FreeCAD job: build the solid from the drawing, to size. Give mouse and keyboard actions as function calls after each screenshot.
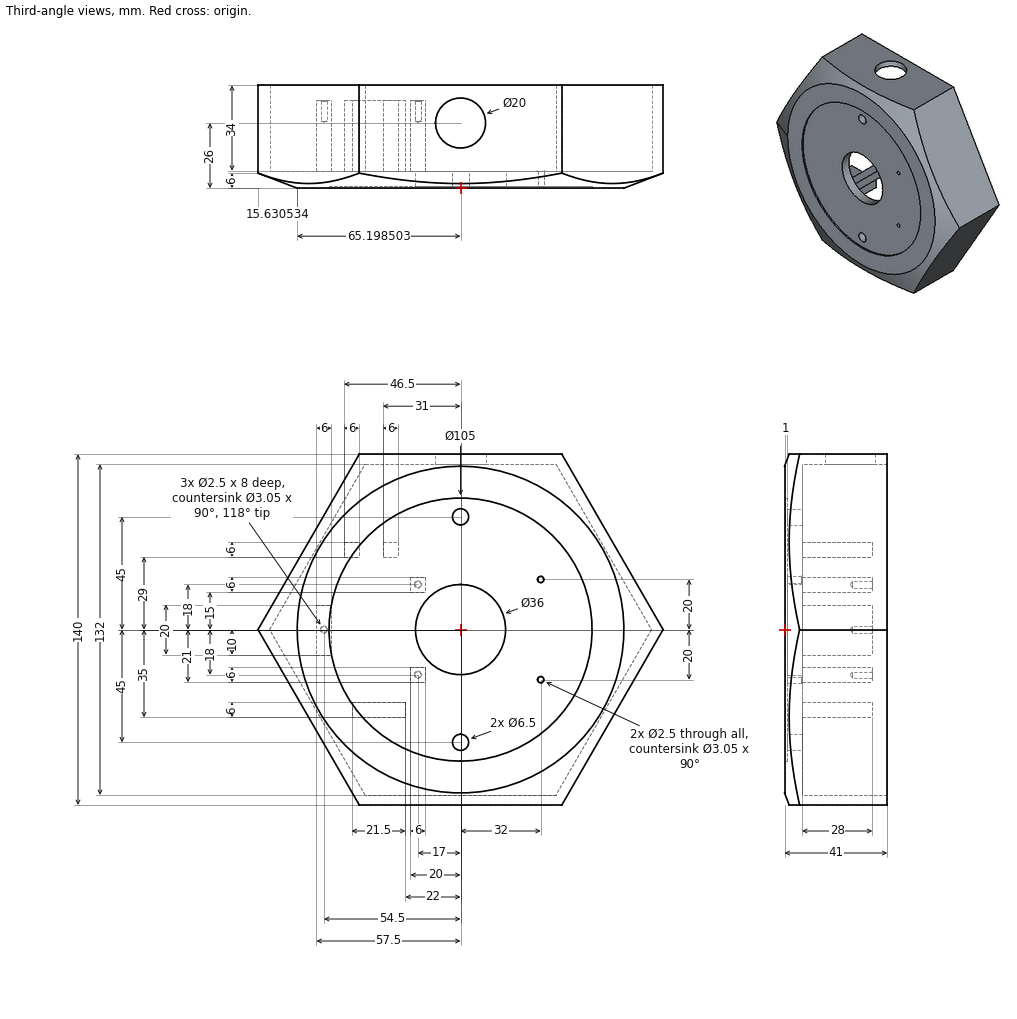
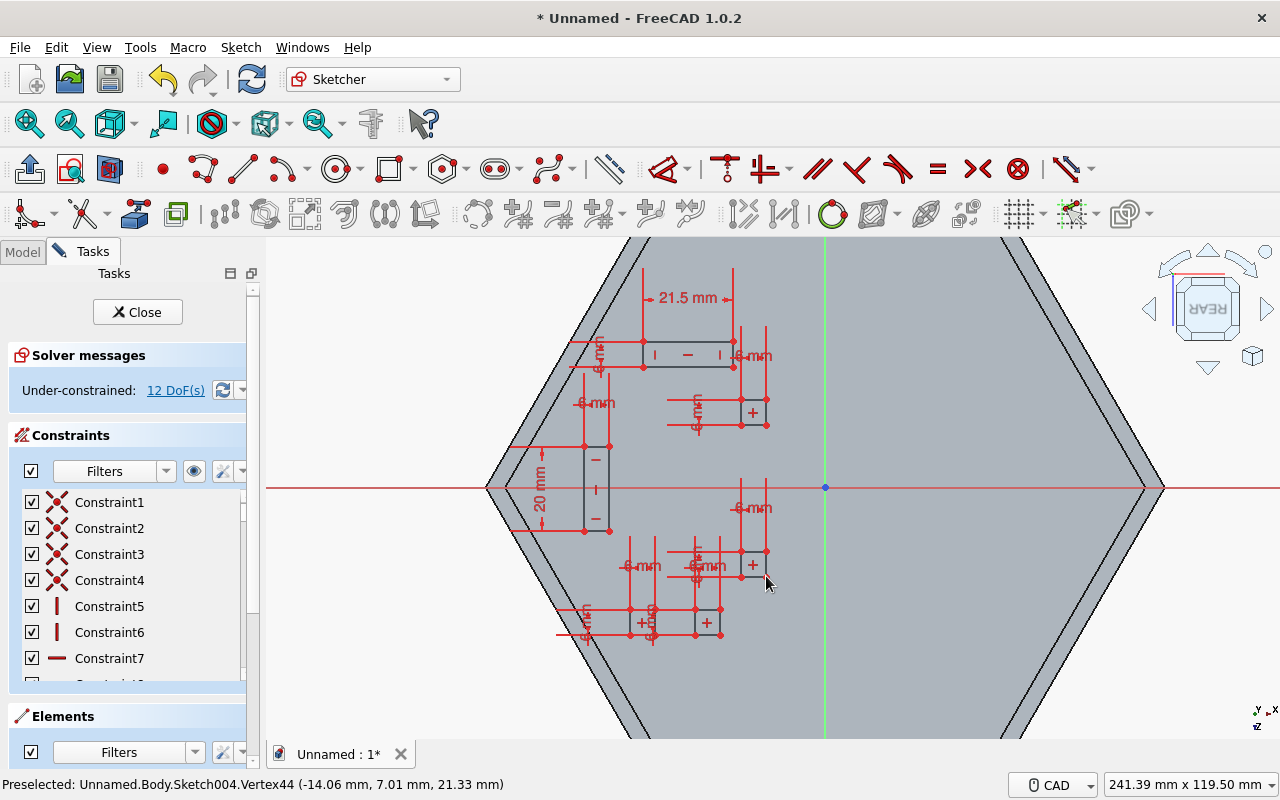
click(643, 342)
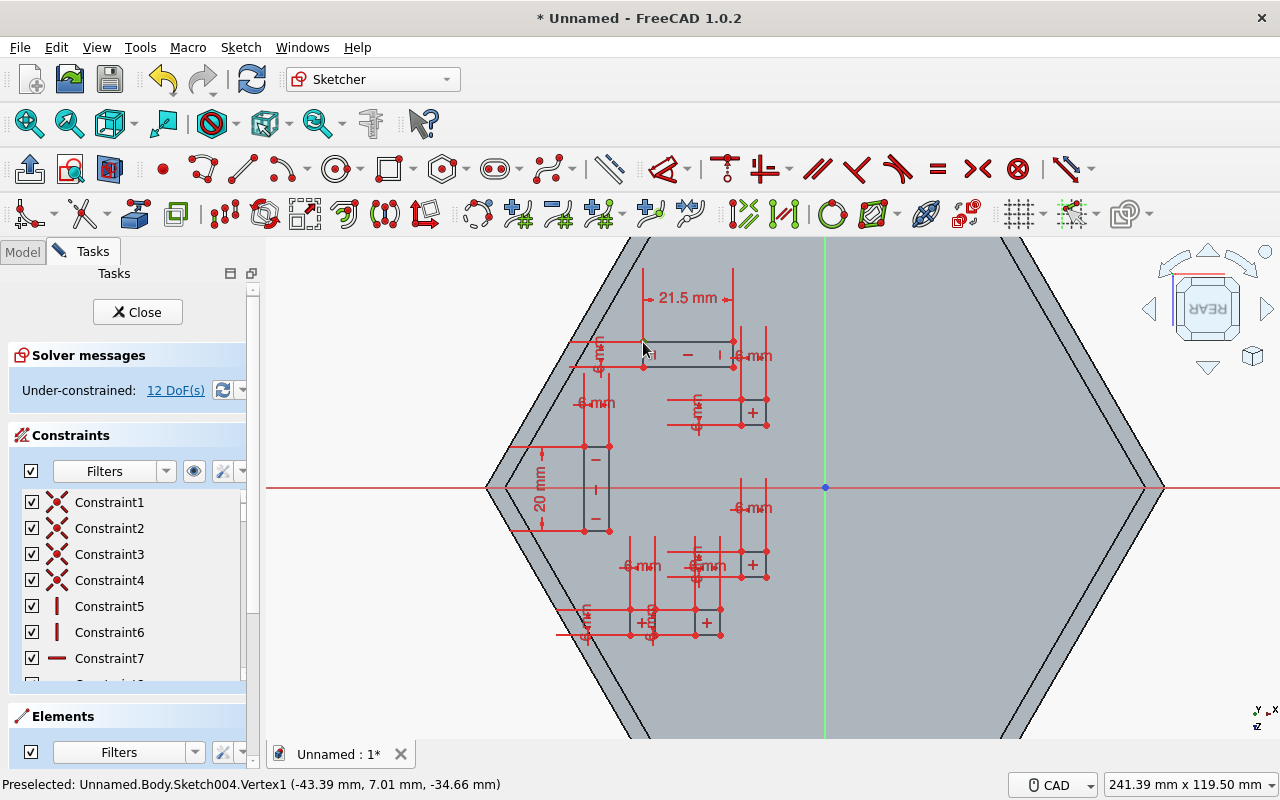
key(i)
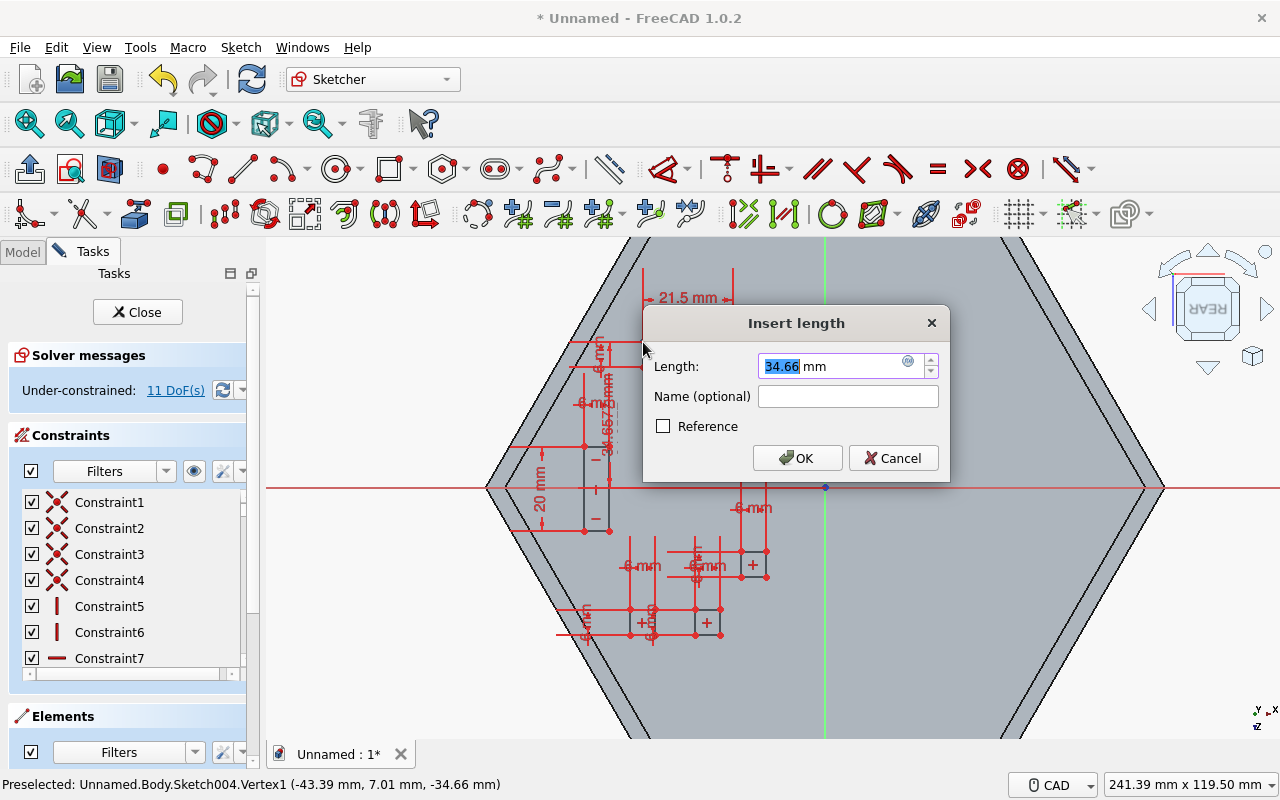
text(35)
key(Return)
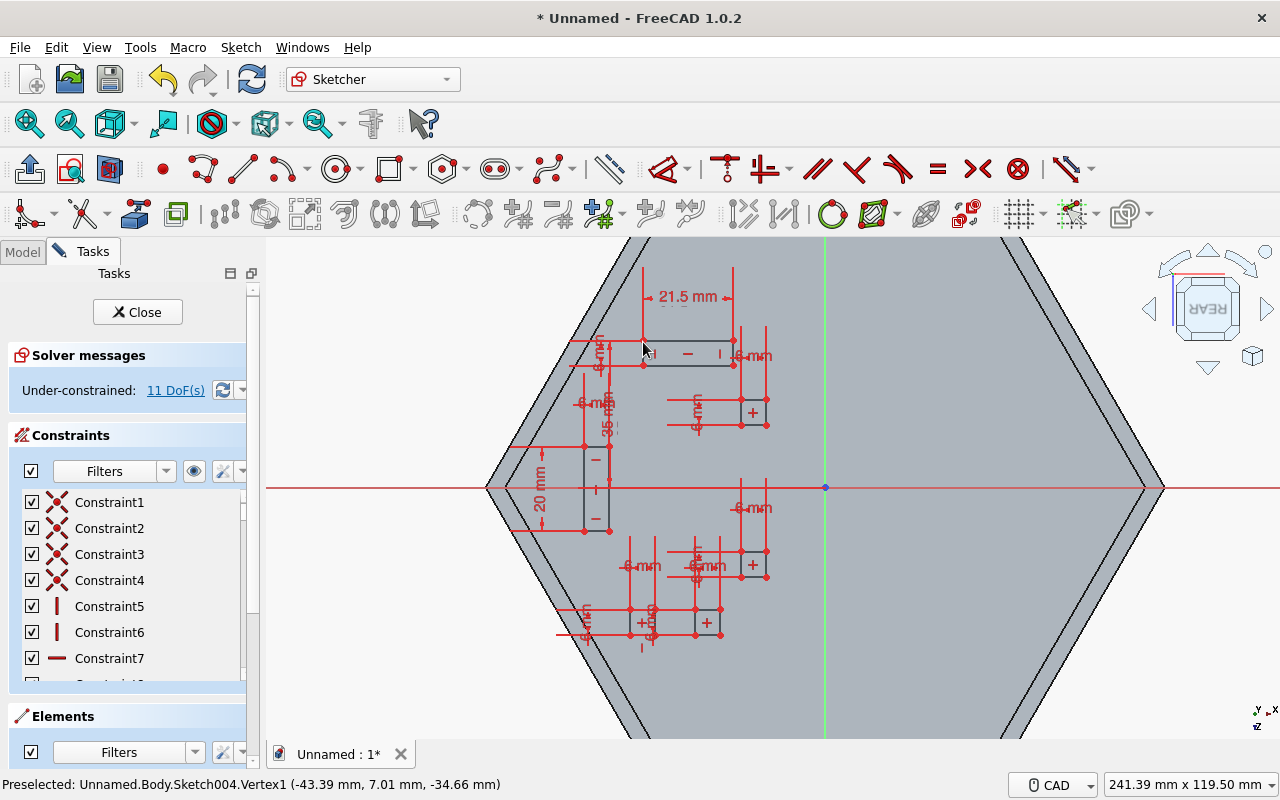
click(733, 366)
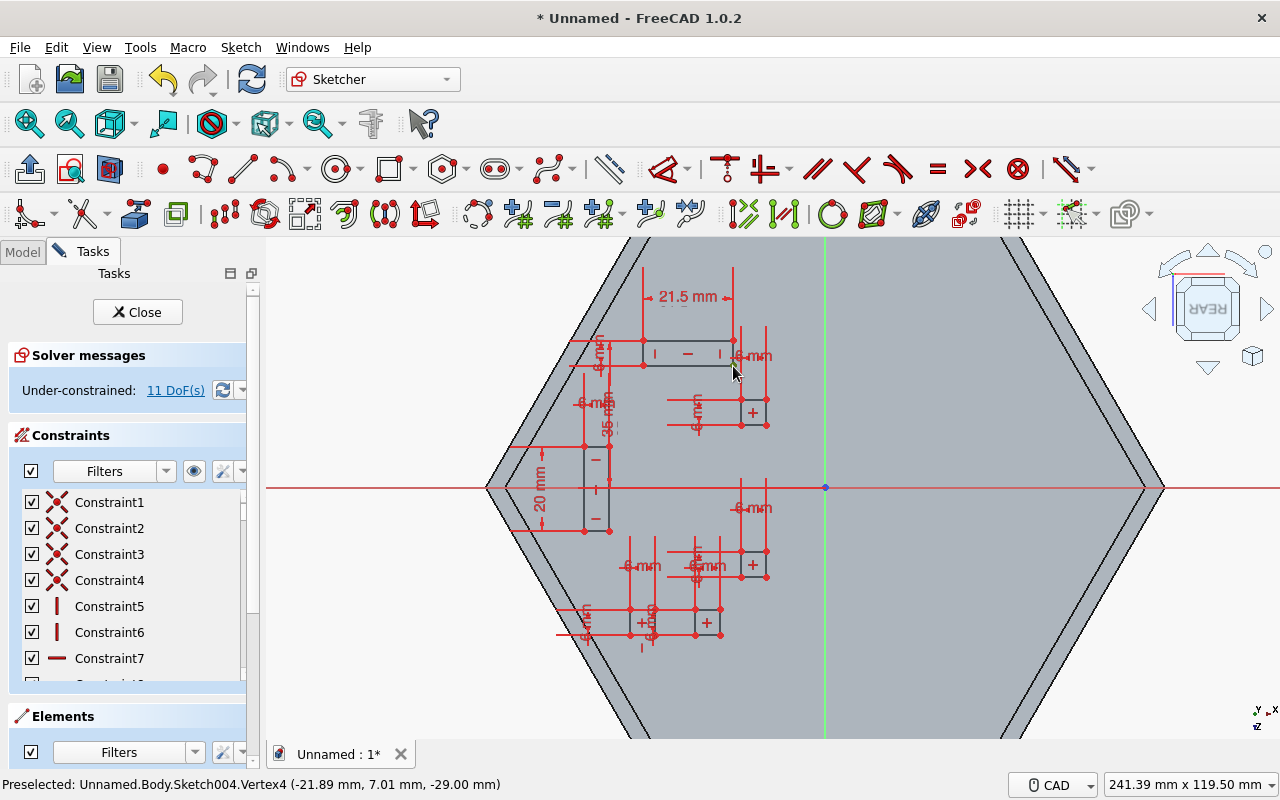
key(l)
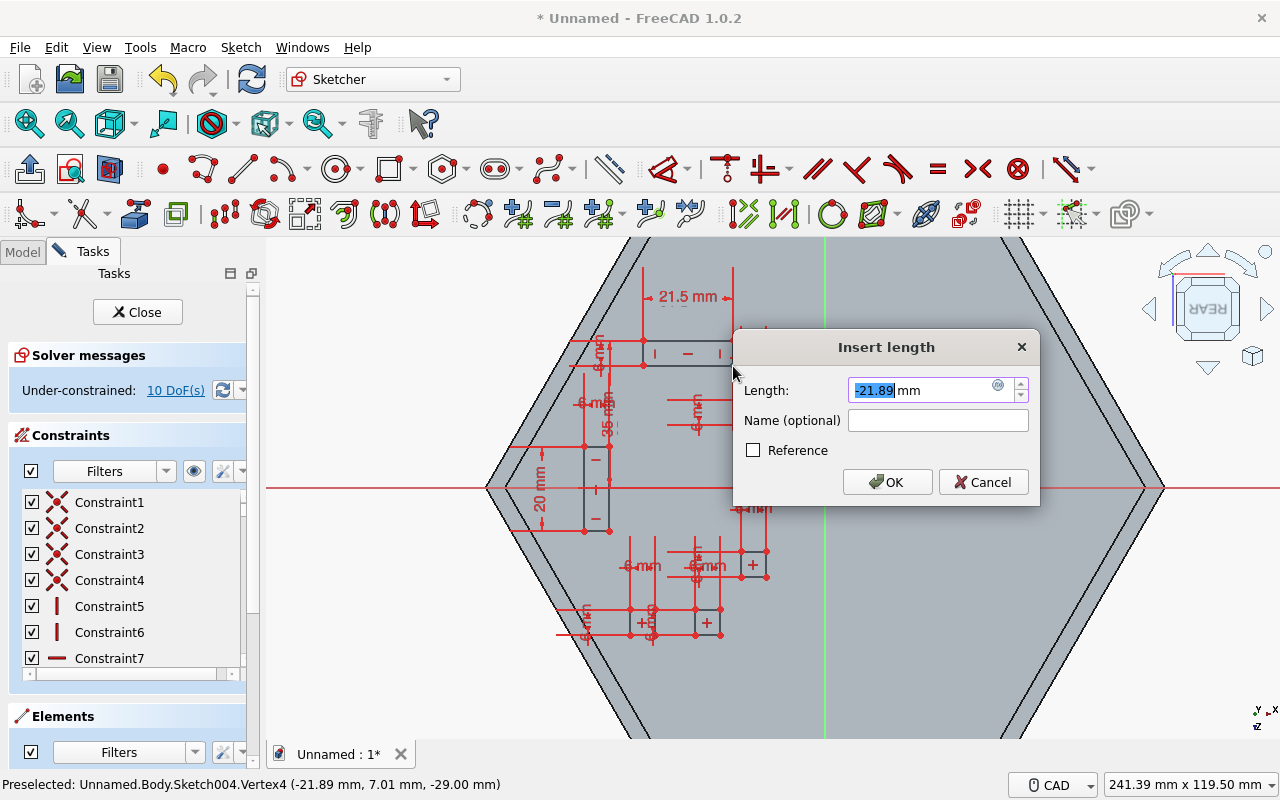
text(-22)
key(Return)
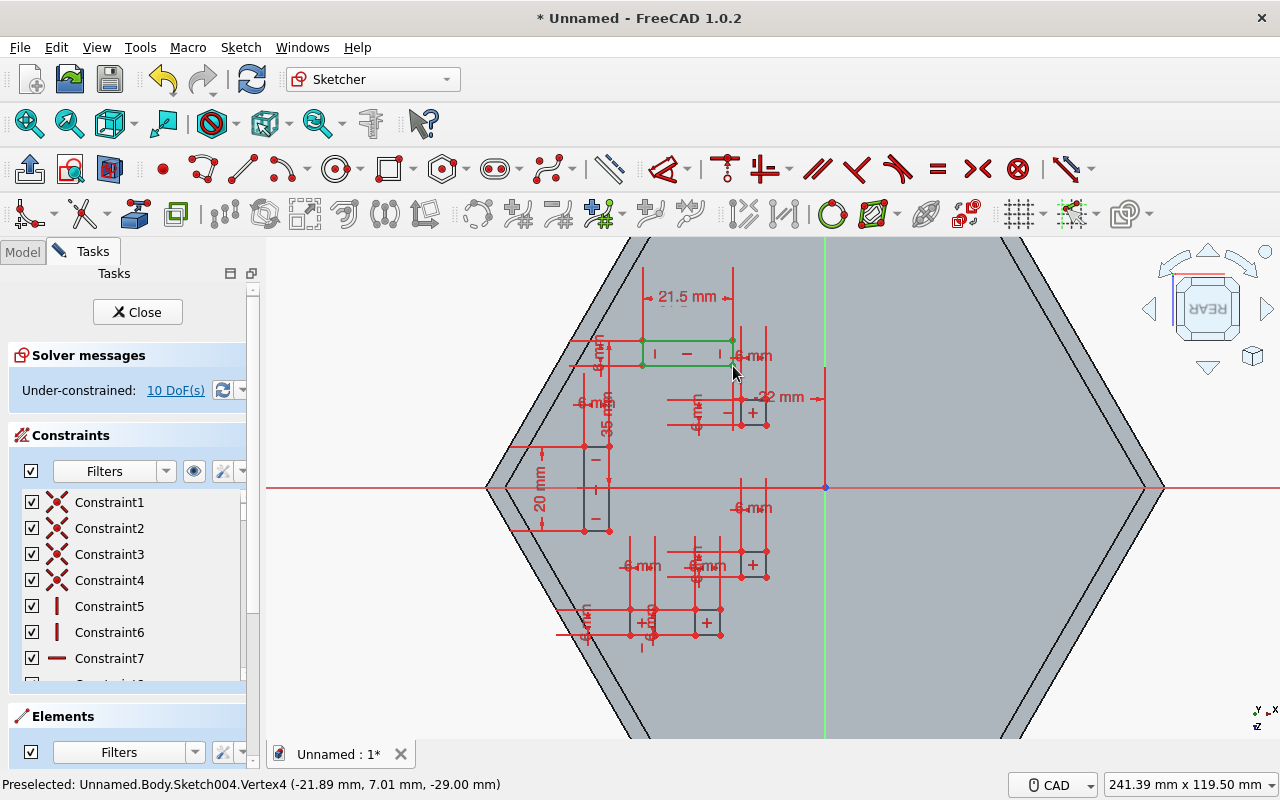
click(584, 447)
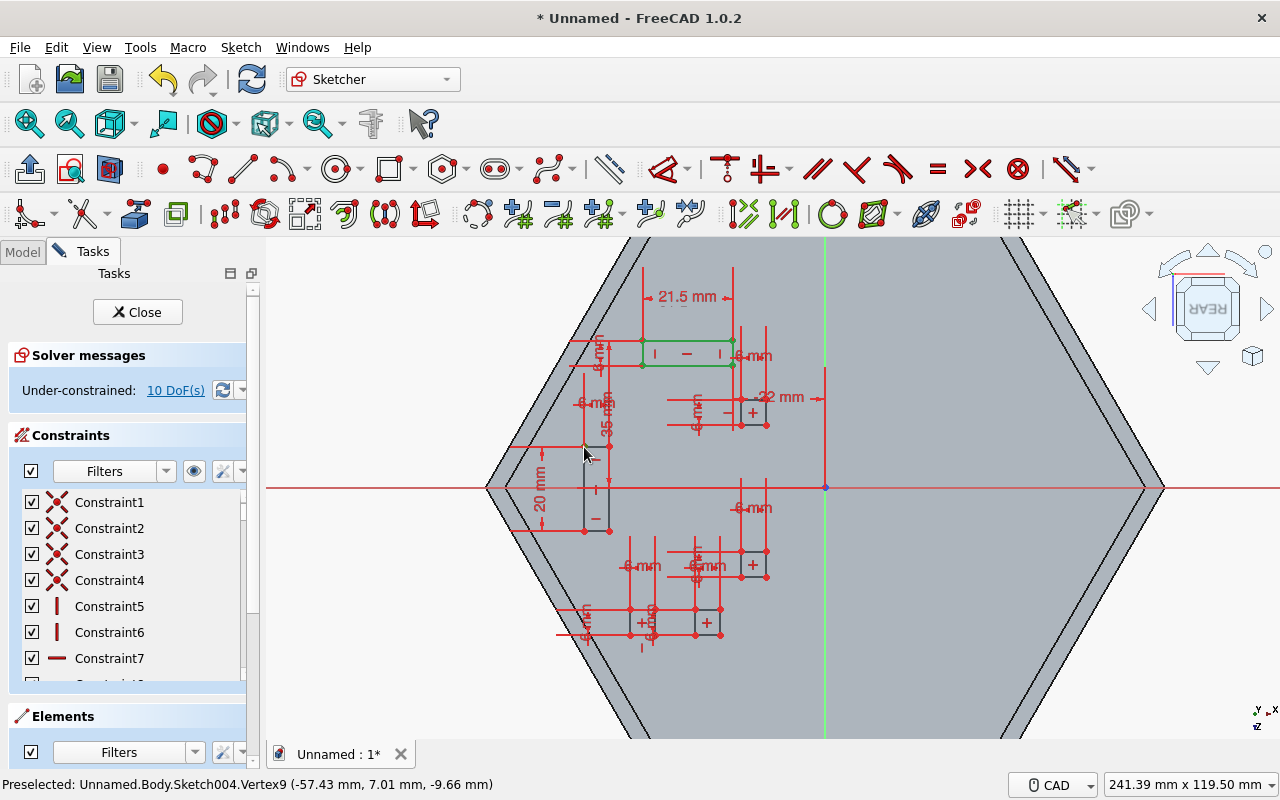
key(i)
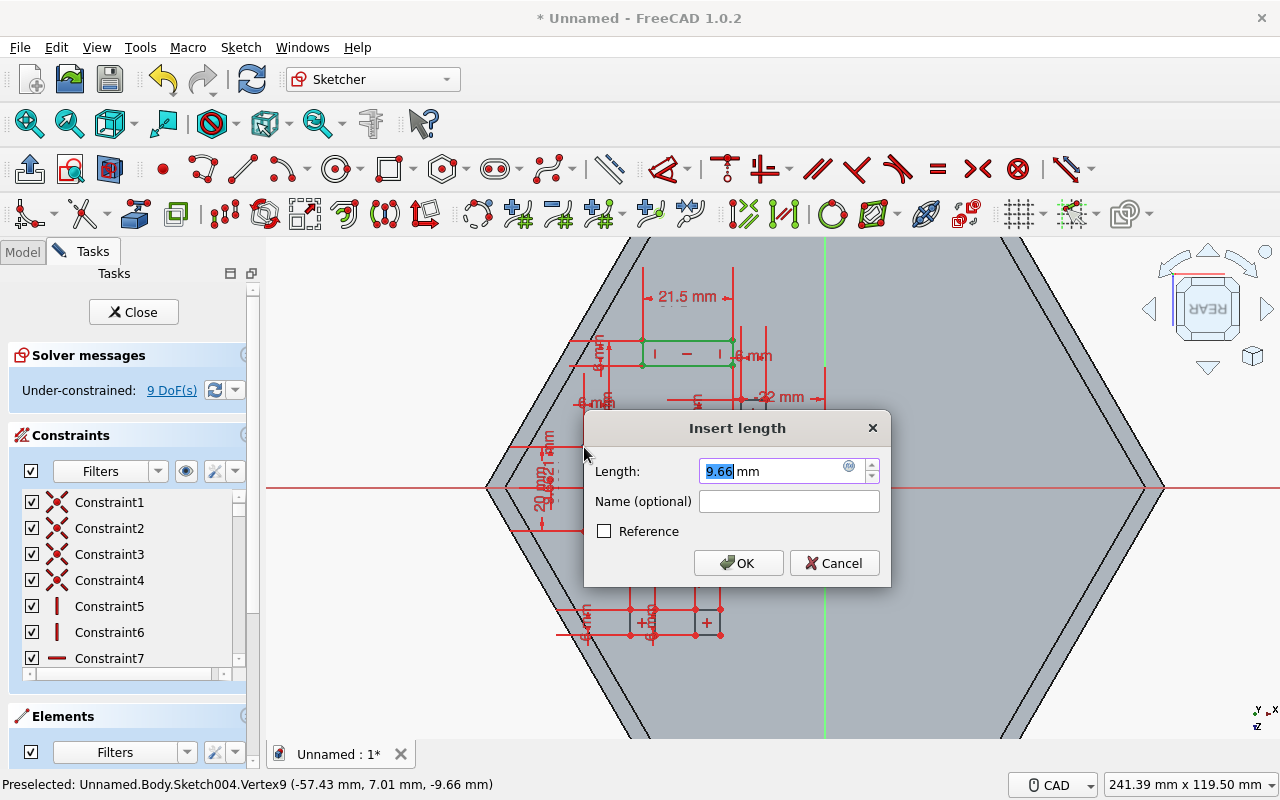
text(10)
key(Return)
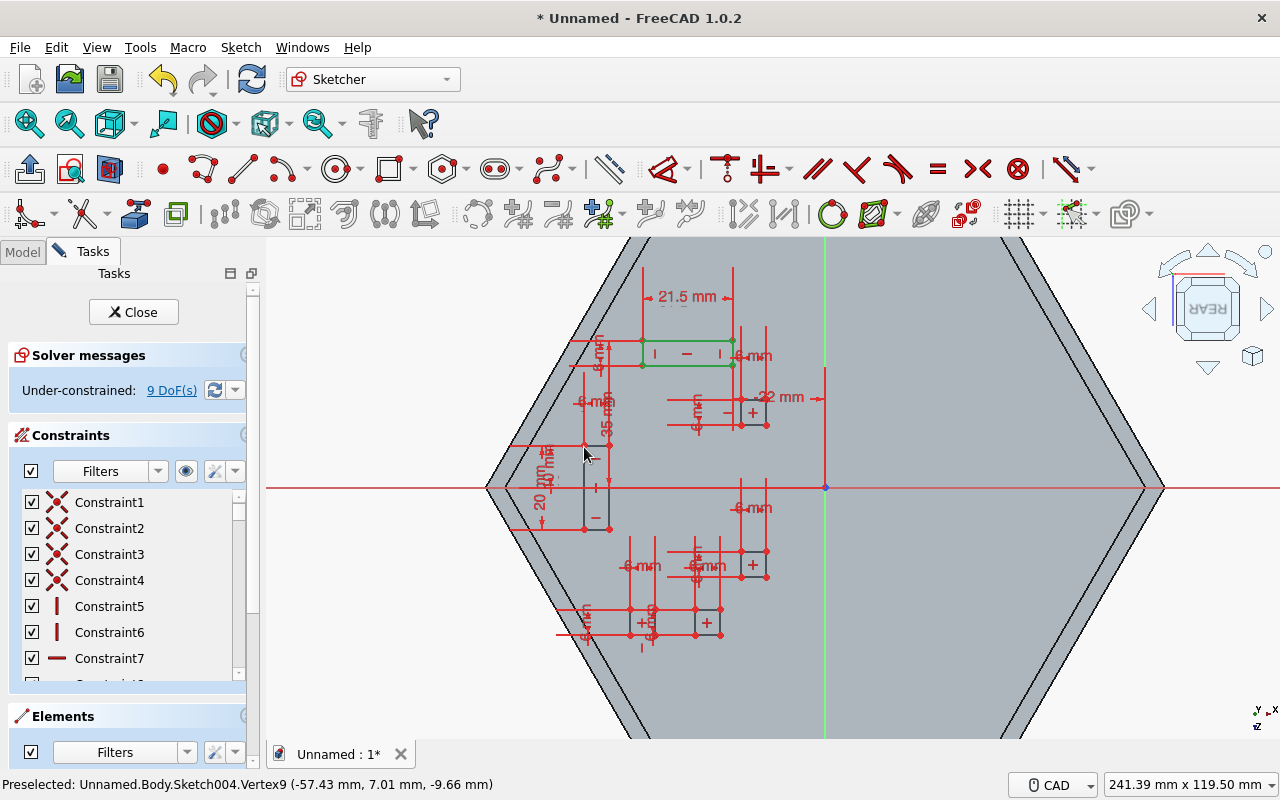
click(630, 610)